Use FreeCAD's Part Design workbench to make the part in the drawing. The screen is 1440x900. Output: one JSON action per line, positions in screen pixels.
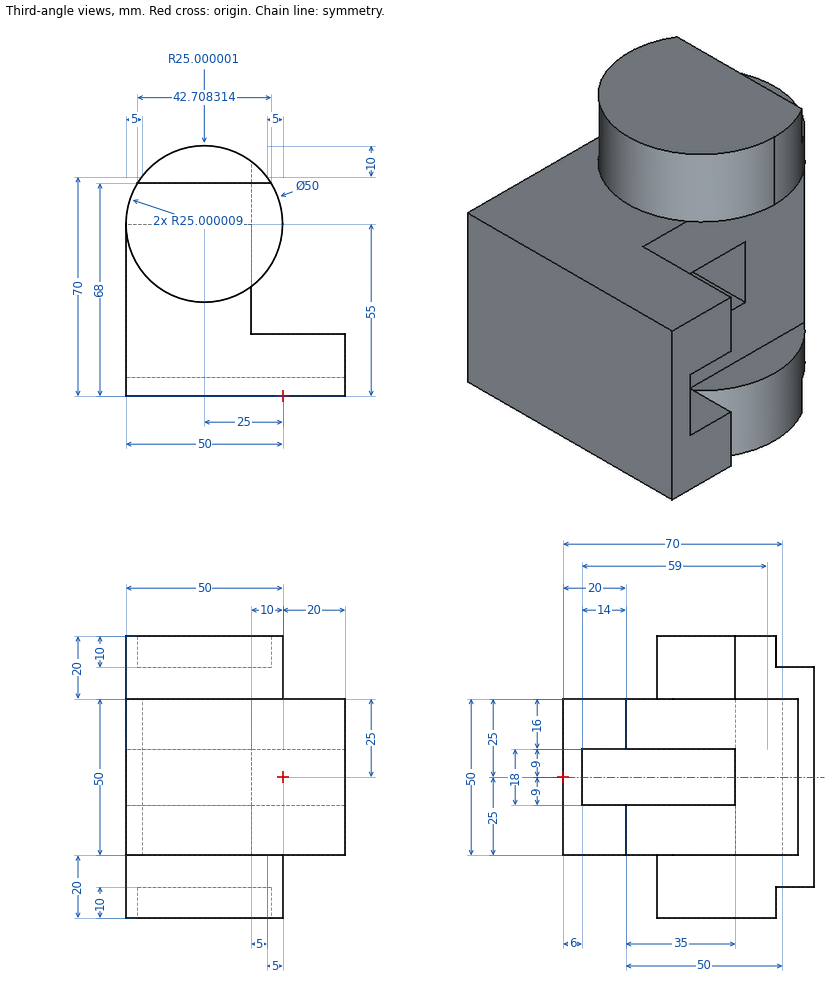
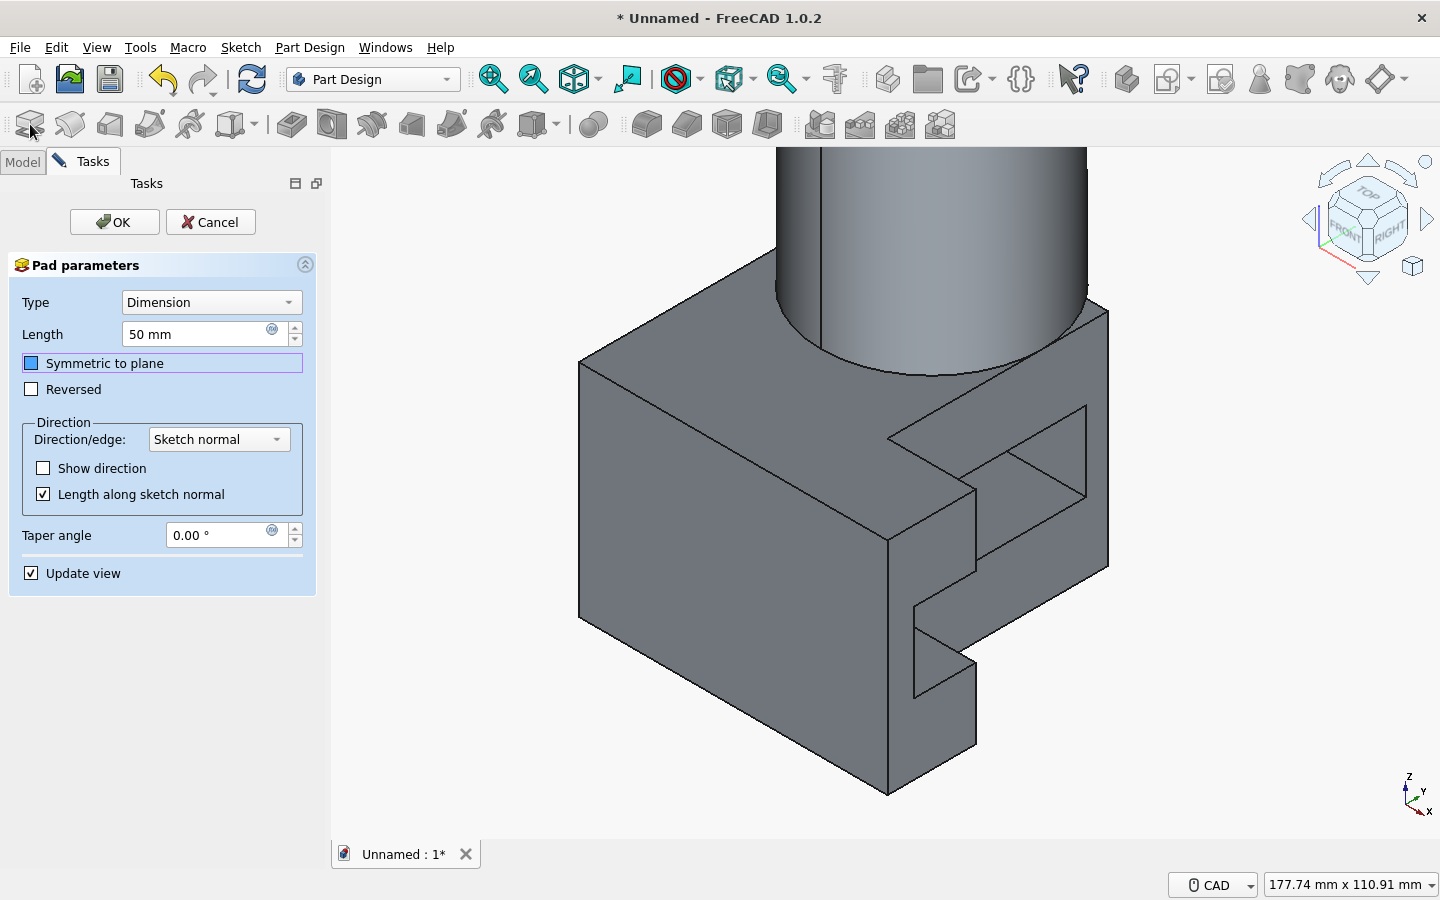
{"action": "left_click", "coordinate": [30, 389]}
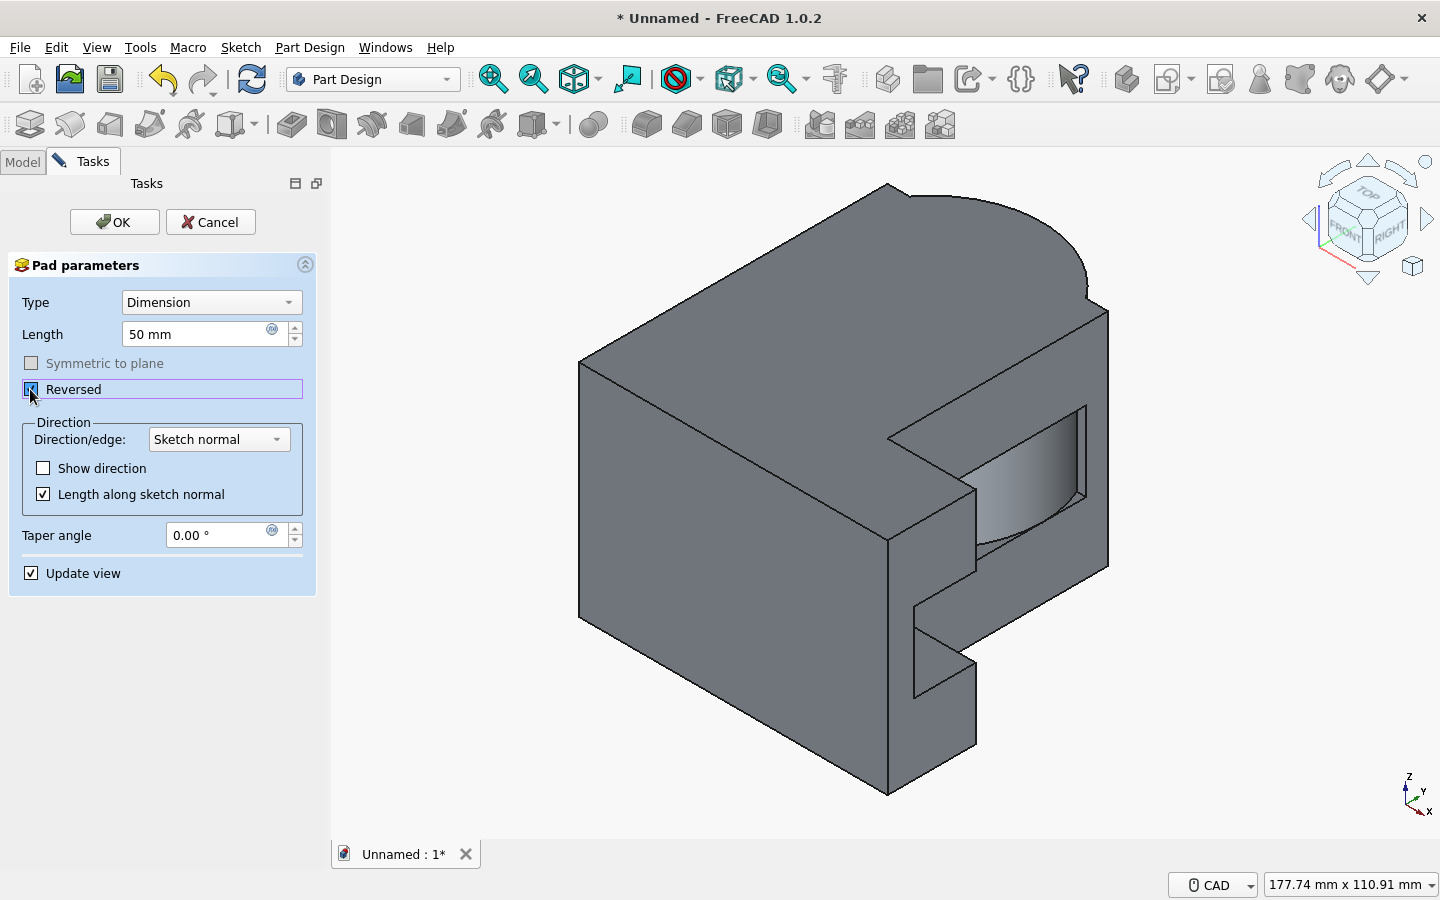
{"action": "left_click", "coordinate": [115, 222]}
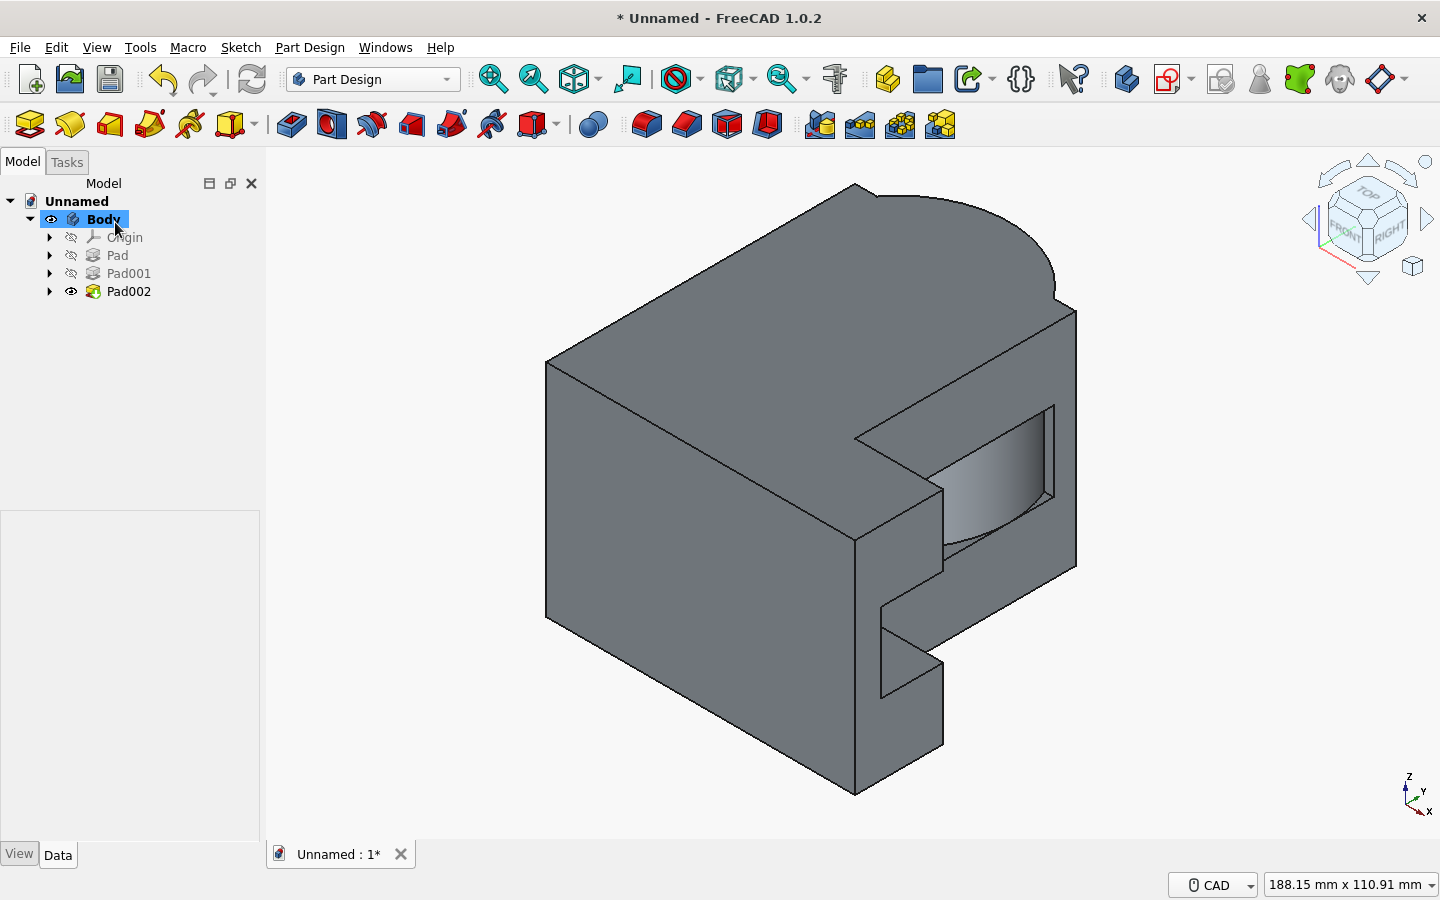
{"action": "left_click", "coordinate": [883, 294]}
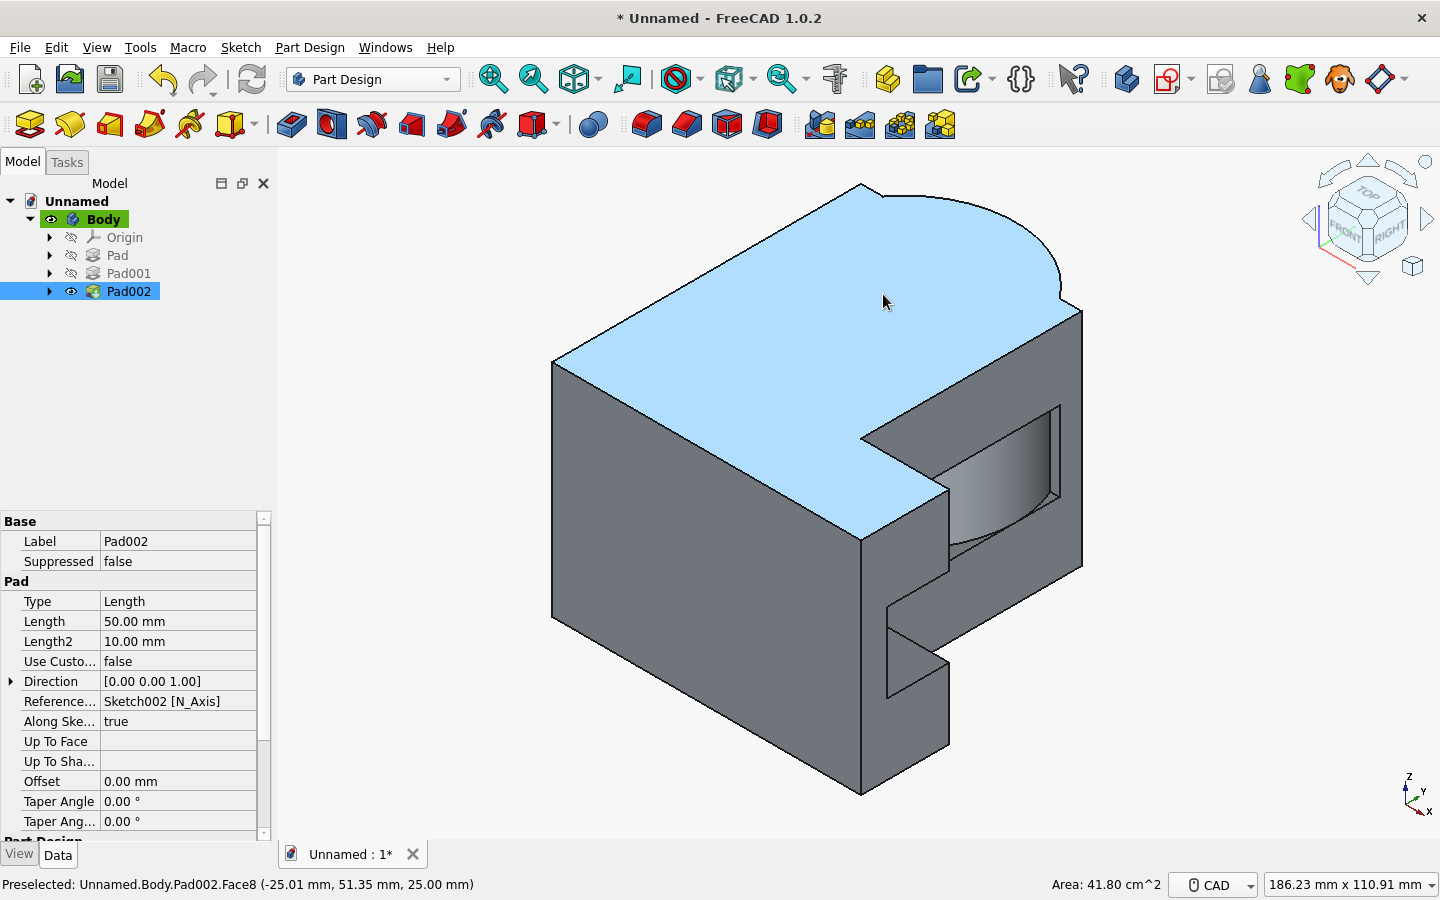
{"action": "left_click", "coordinate": [1168, 80]}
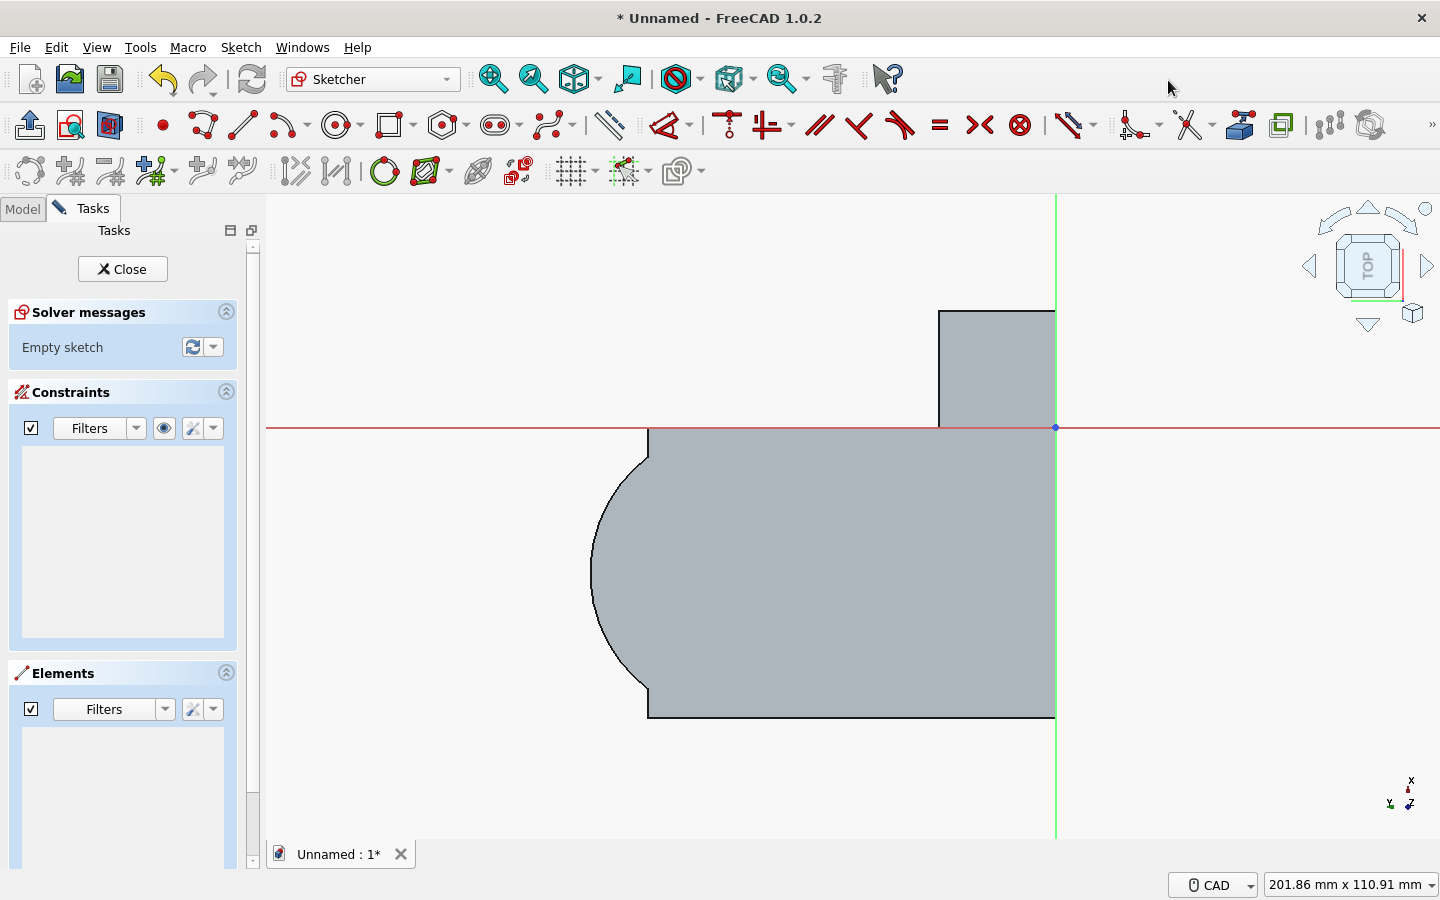
{"action": "scroll", "coordinate": [989, 688], "scroll_direction": "up", "scroll_amount": 2}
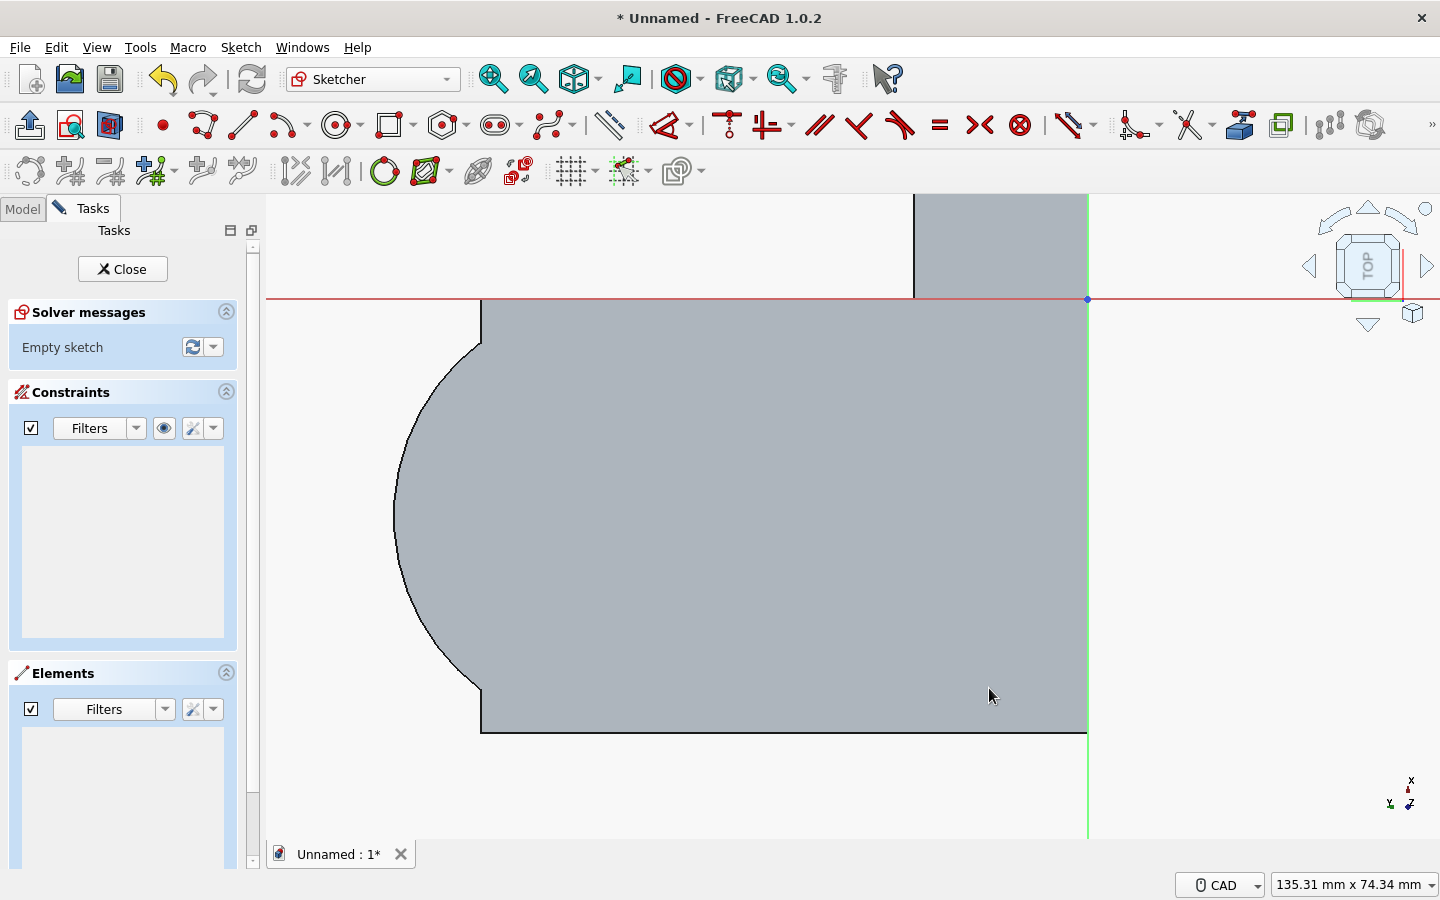
{"action": "left_click", "coordinate": [204, 126]}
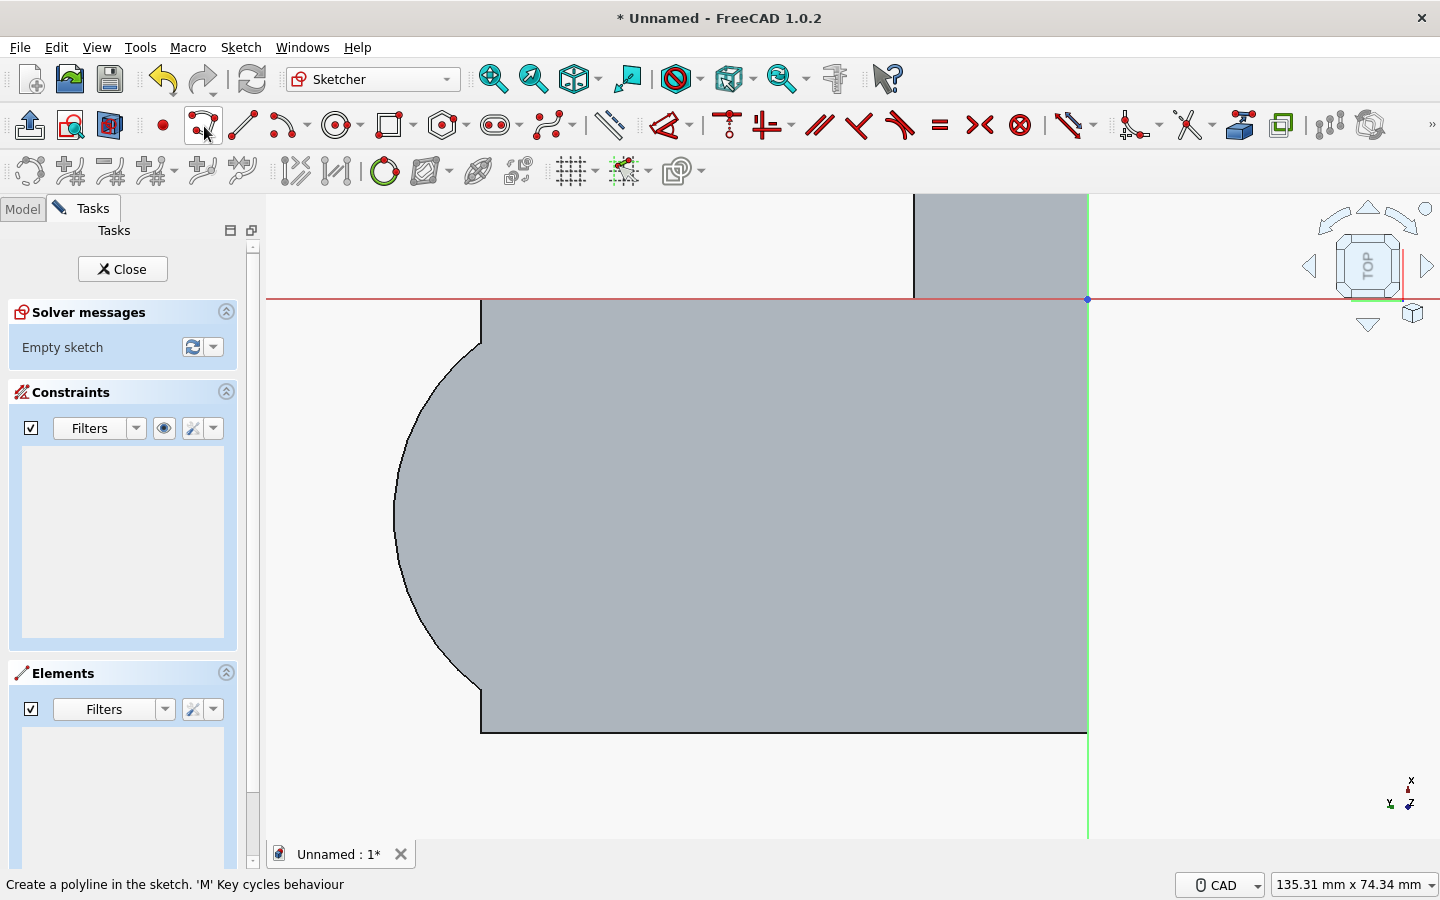
{"action": "left_click", "coordinate": [481, 690]}
{"action": "left_click", "coordinate": [481, 733]}
{"action": "left_click", "coordinate": [611, 733]}
{"action": "right_click", "coordinate": [611, 733]}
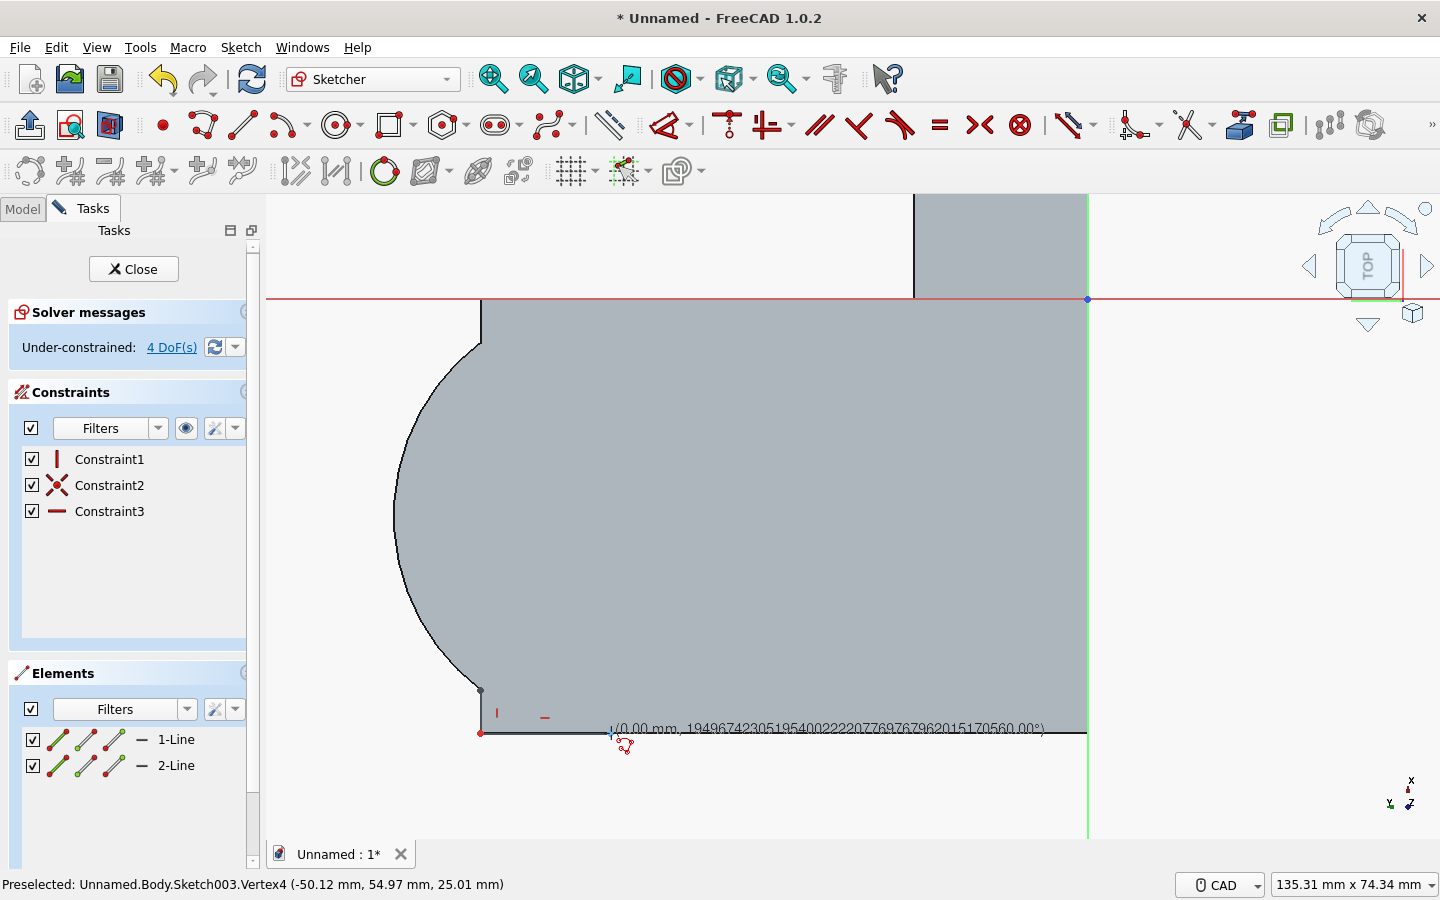
{"action": "left_click", "coordinate": [310, 126]}